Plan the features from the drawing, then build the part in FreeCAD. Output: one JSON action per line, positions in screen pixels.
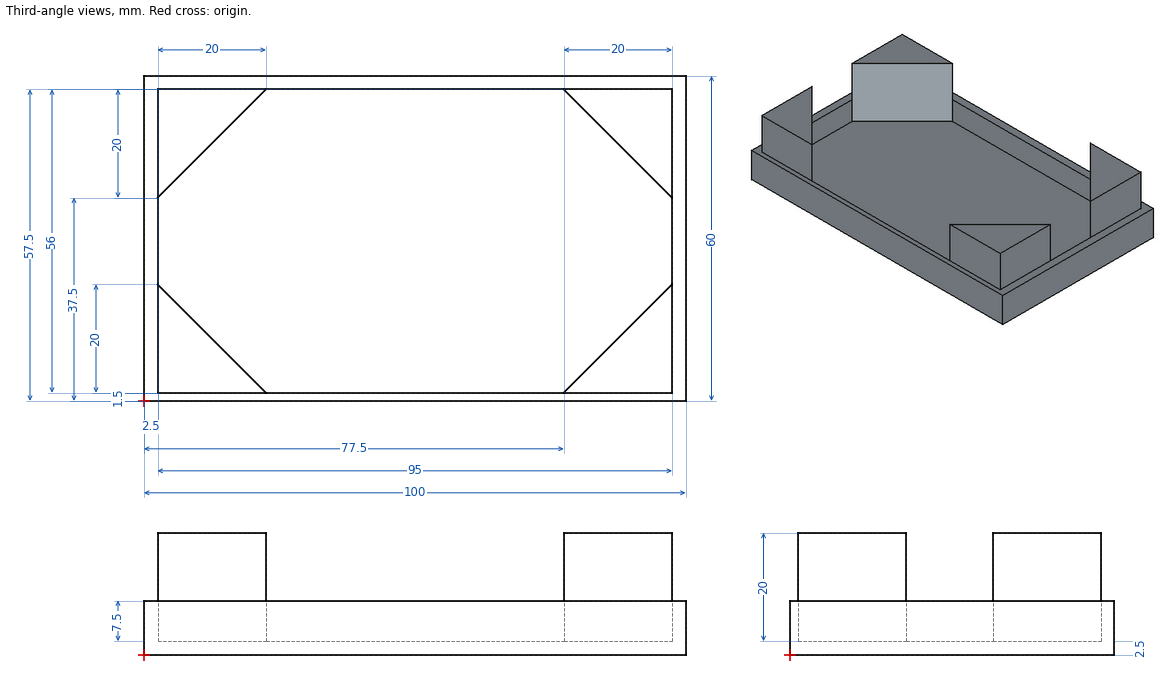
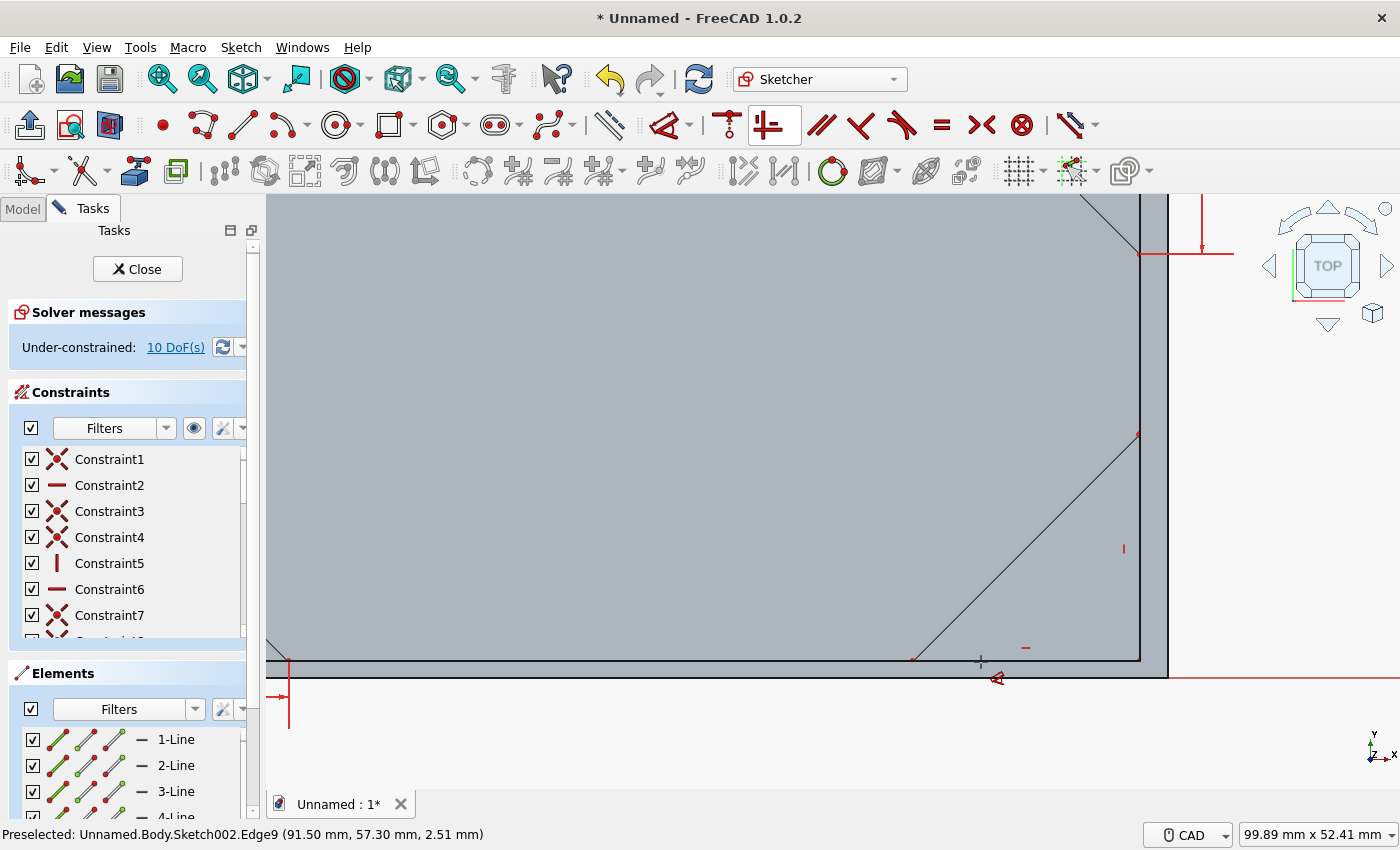
{"action": "left_click", "coordinate": [981, 662]}
{"action": "left_click", "coordinate": [1026, 696]}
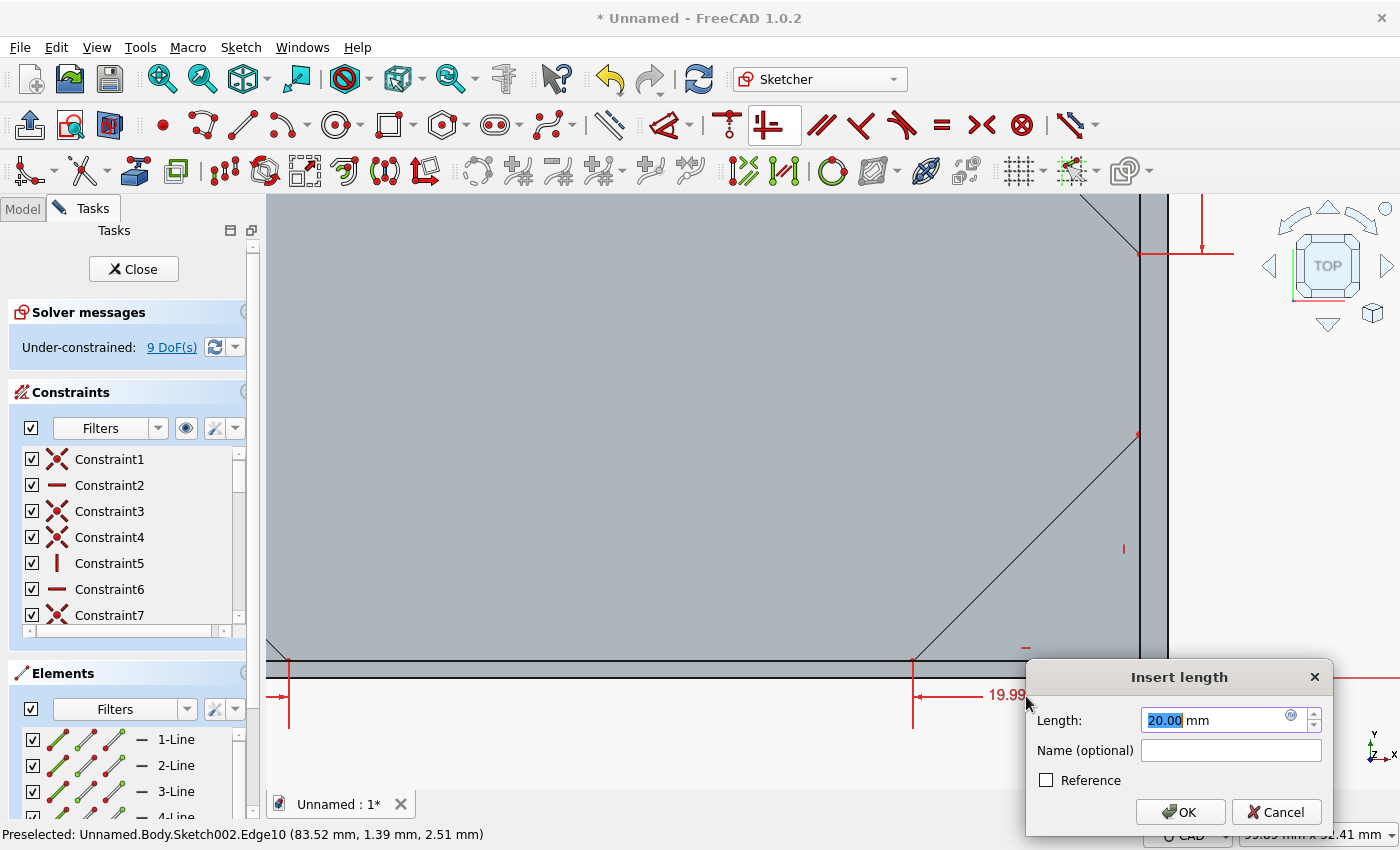
{"action": "type", "text": "20"}
{"action": "key", "text": "Return"}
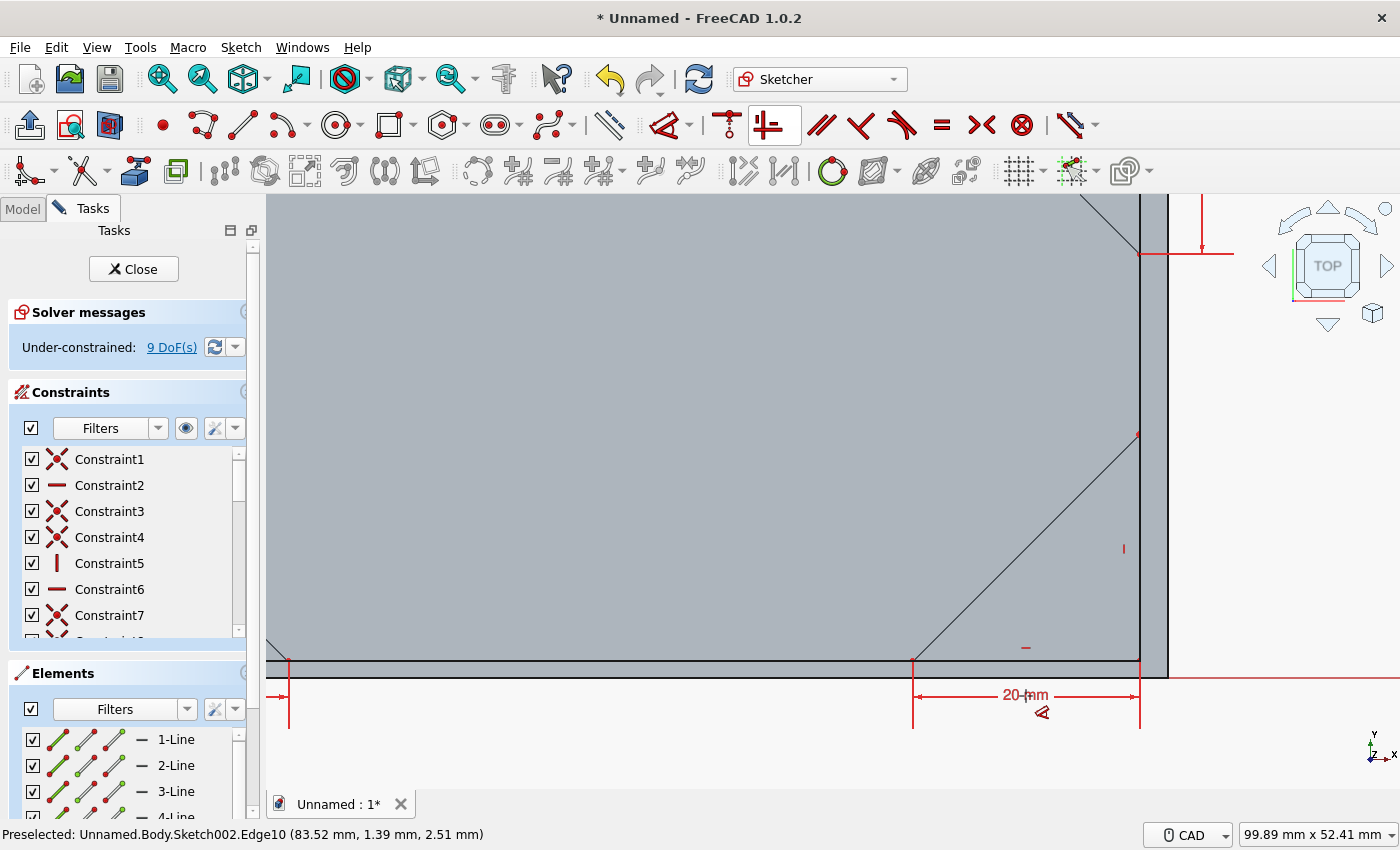
{"action": "left_click", "coordinate": [1140, 594]}
{"action": "left_click", "coordinate": [1174, 548]}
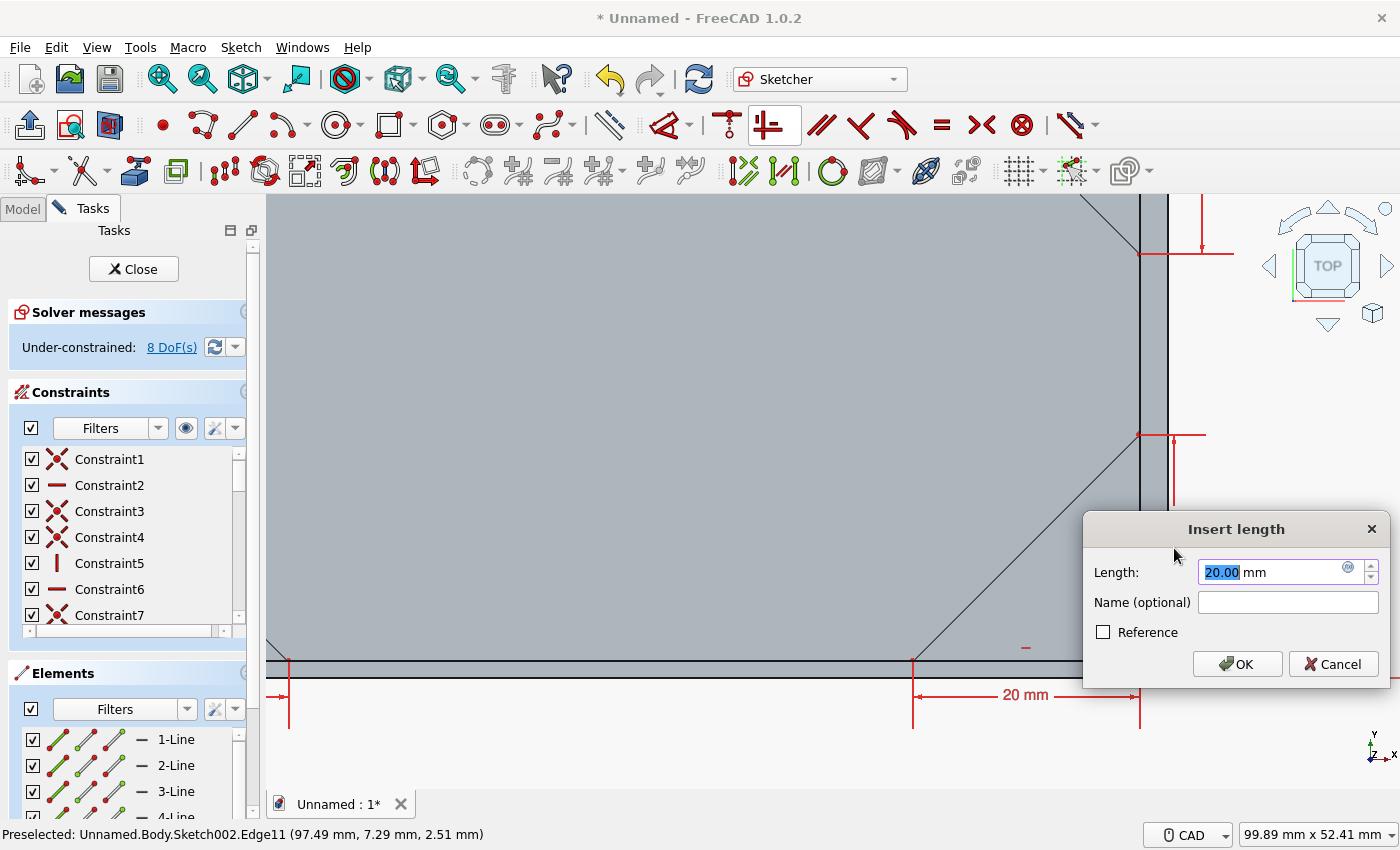
{"action": "type", "text": "20"}
{"action": "key", "text": "Return"}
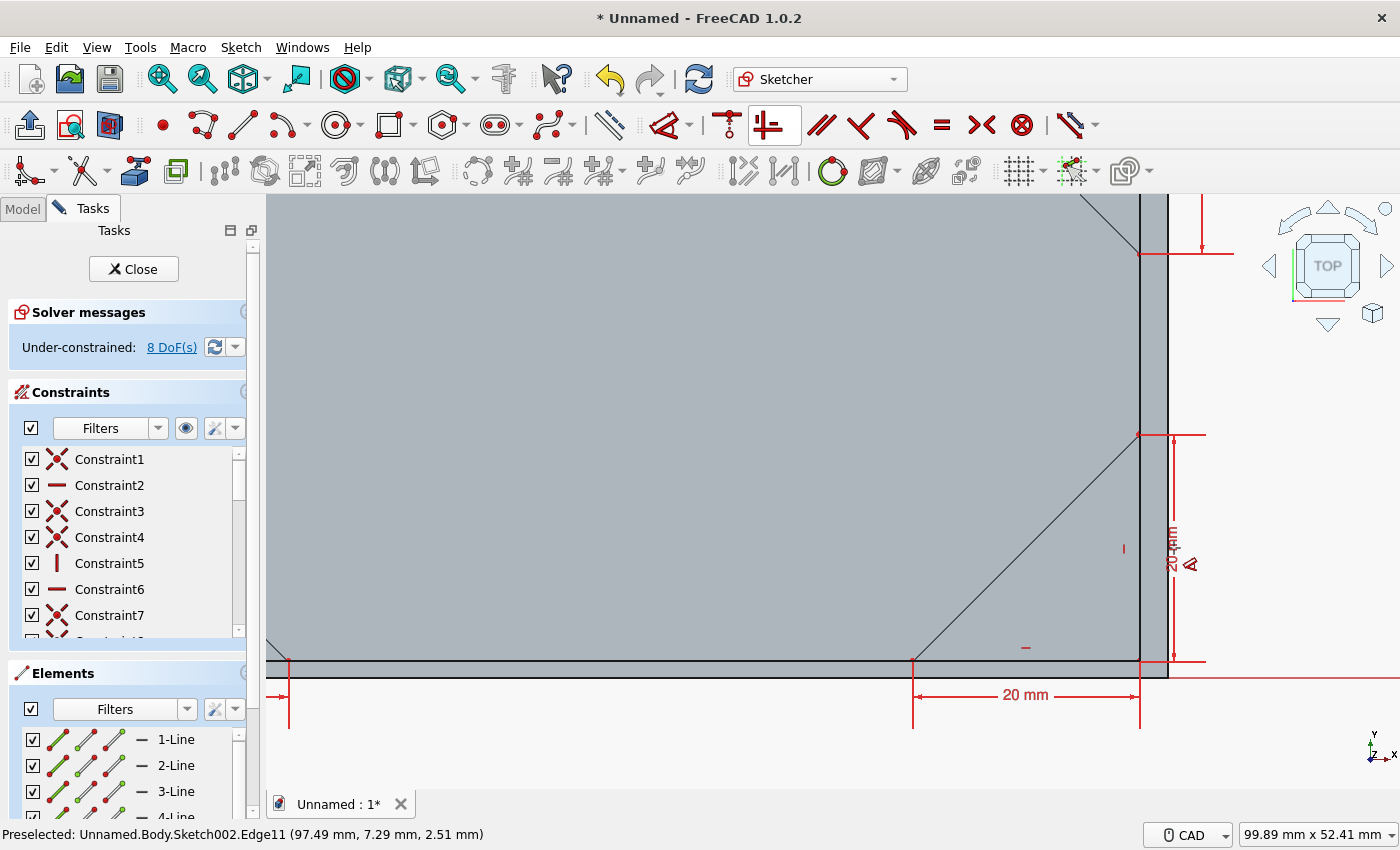
{"action": "scroll", "coordinate": [981, 662], "scroll_direction": "down", "scroll_amount": 3}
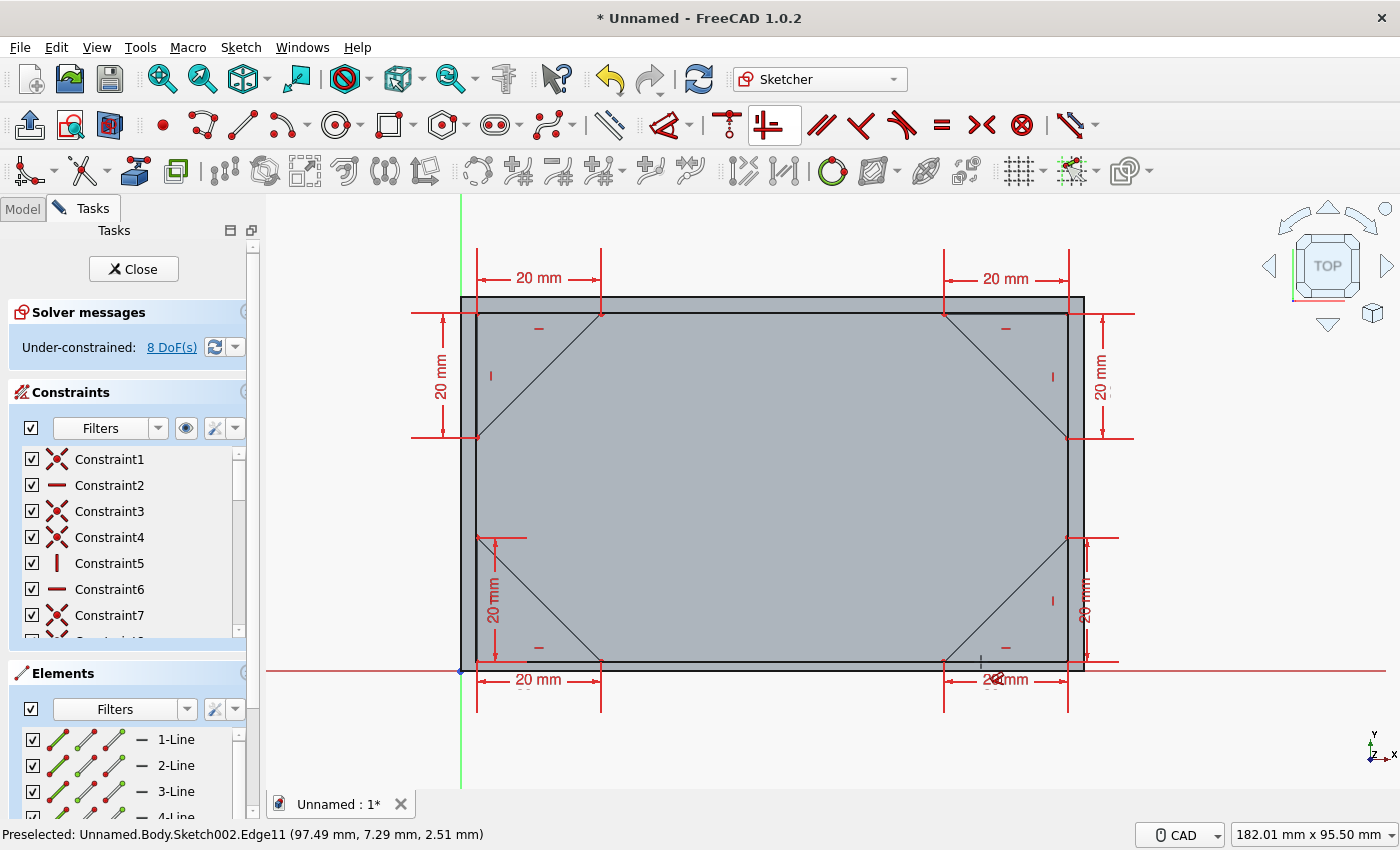
{"action": "scroll", "coordinate": [477, 438], "scroll_direction": "up", "scroll_amount": 5}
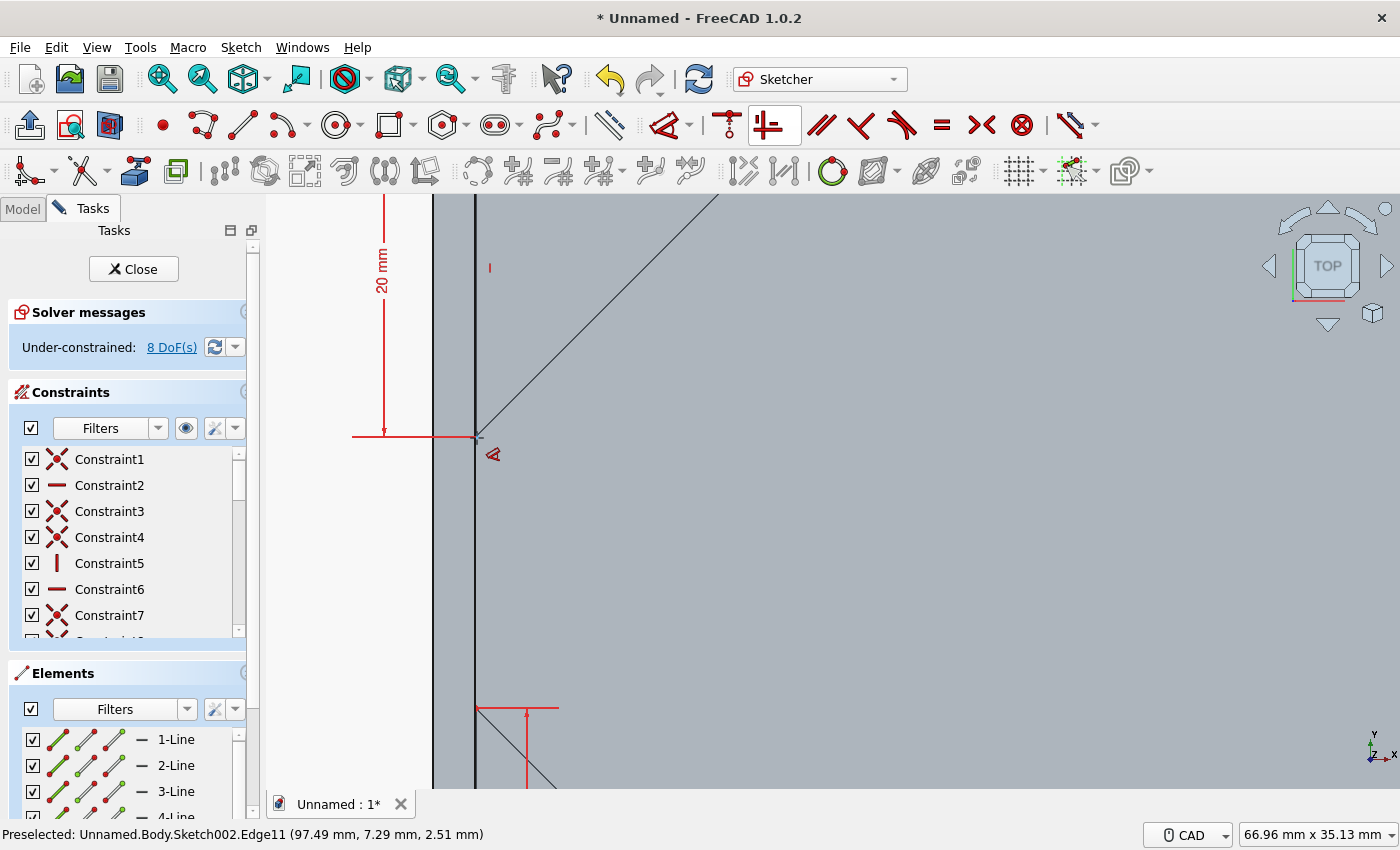
{"action": "left_click", "coordinate": [476, 437]}
{"action": "left_click", "coordinate": [454, 403]}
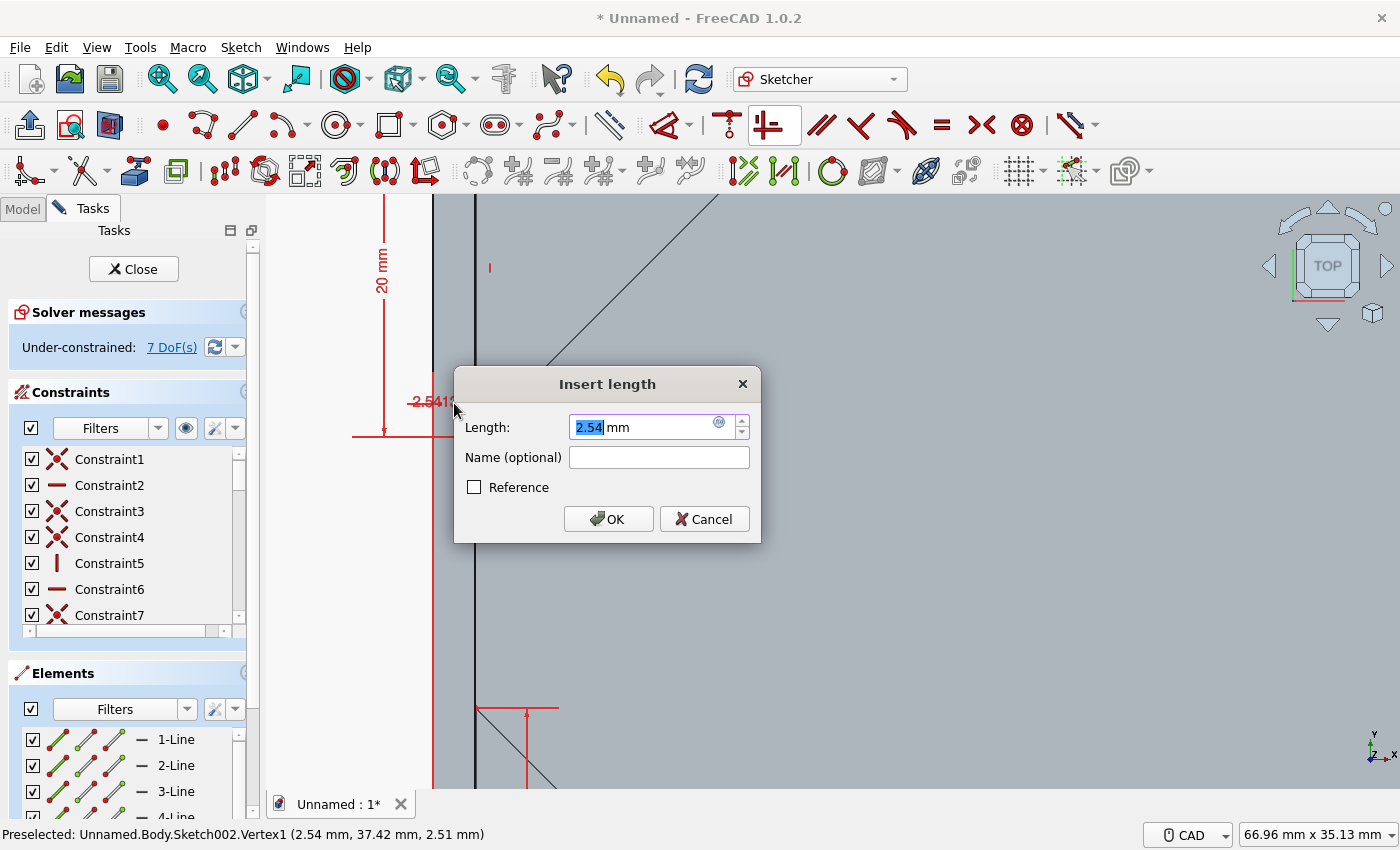
{"action": "type", "text": "2.5"}
{"action": "key", "text": "Return"}